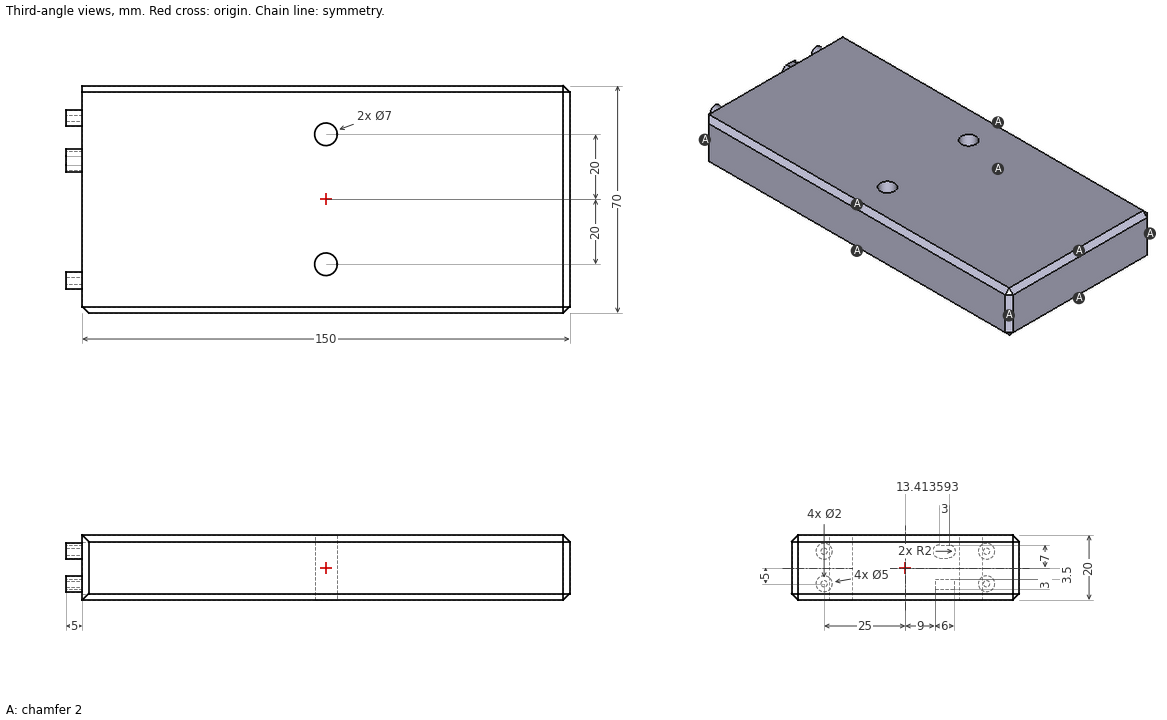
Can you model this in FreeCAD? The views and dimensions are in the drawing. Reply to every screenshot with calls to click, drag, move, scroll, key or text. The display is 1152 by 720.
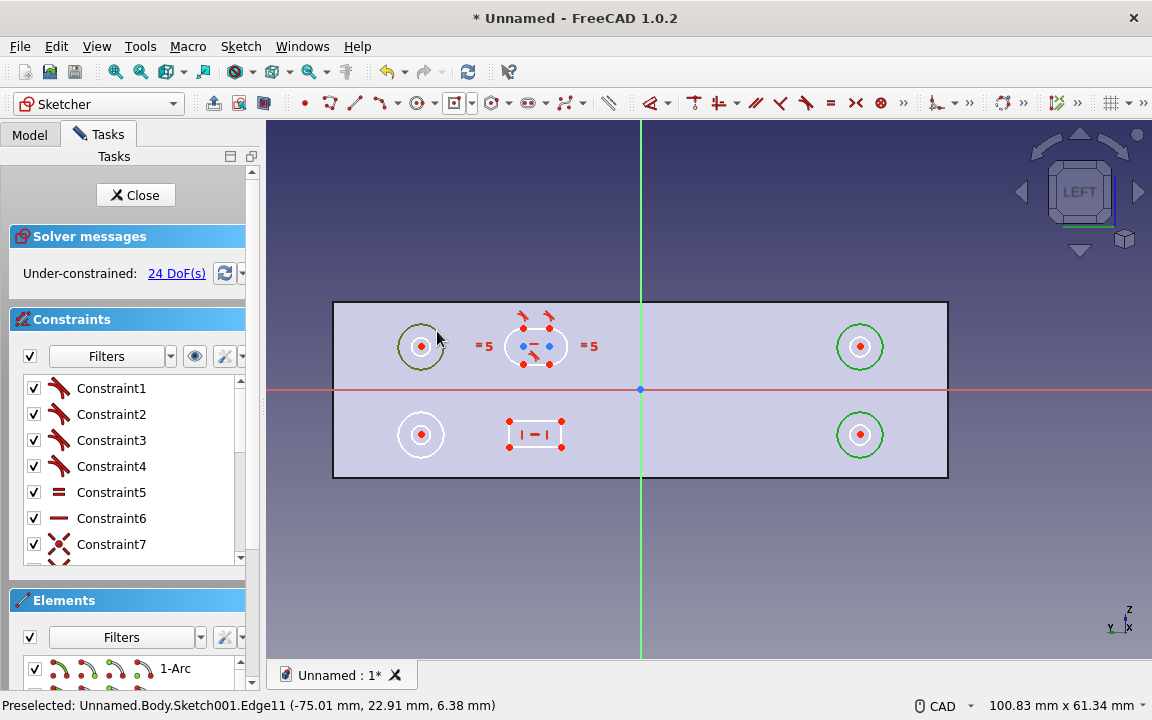
click(437, 419)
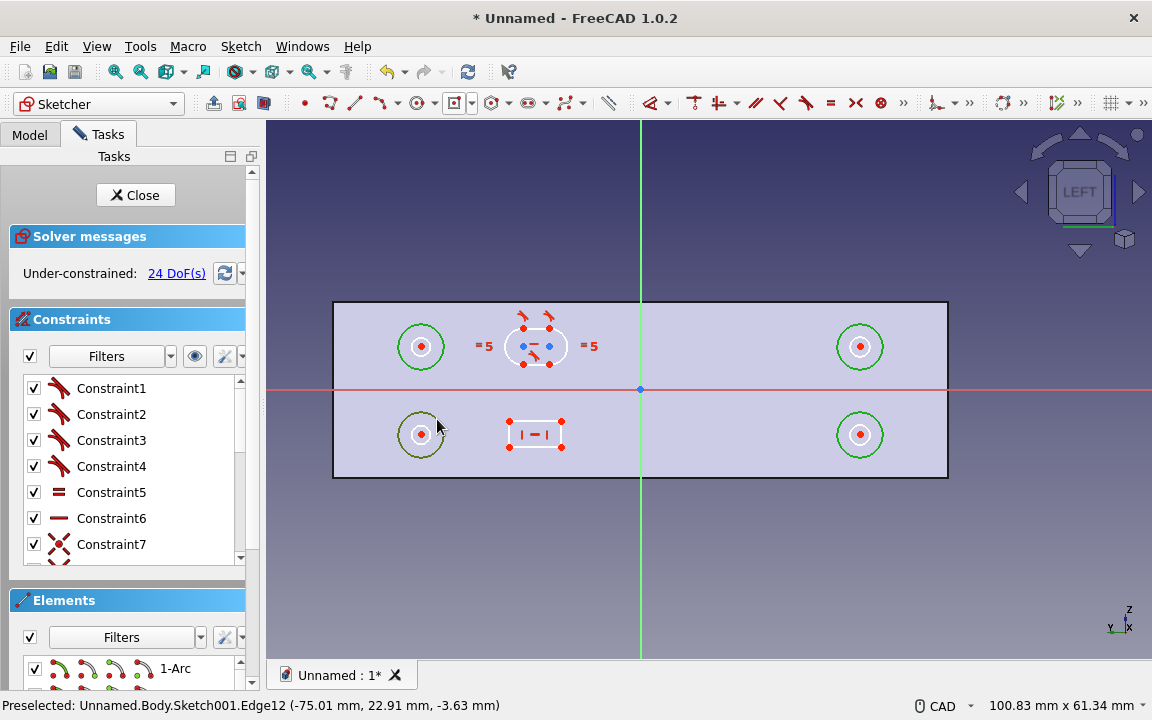
click(831, 104)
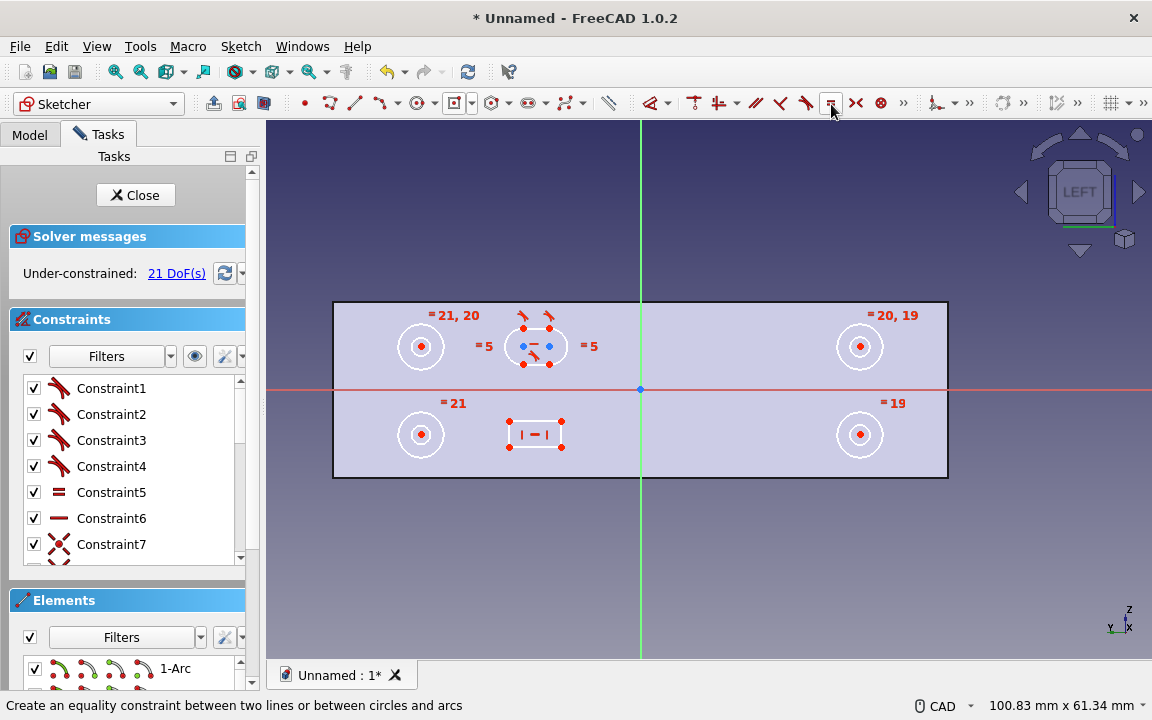
scroll(867, 428, up, 2)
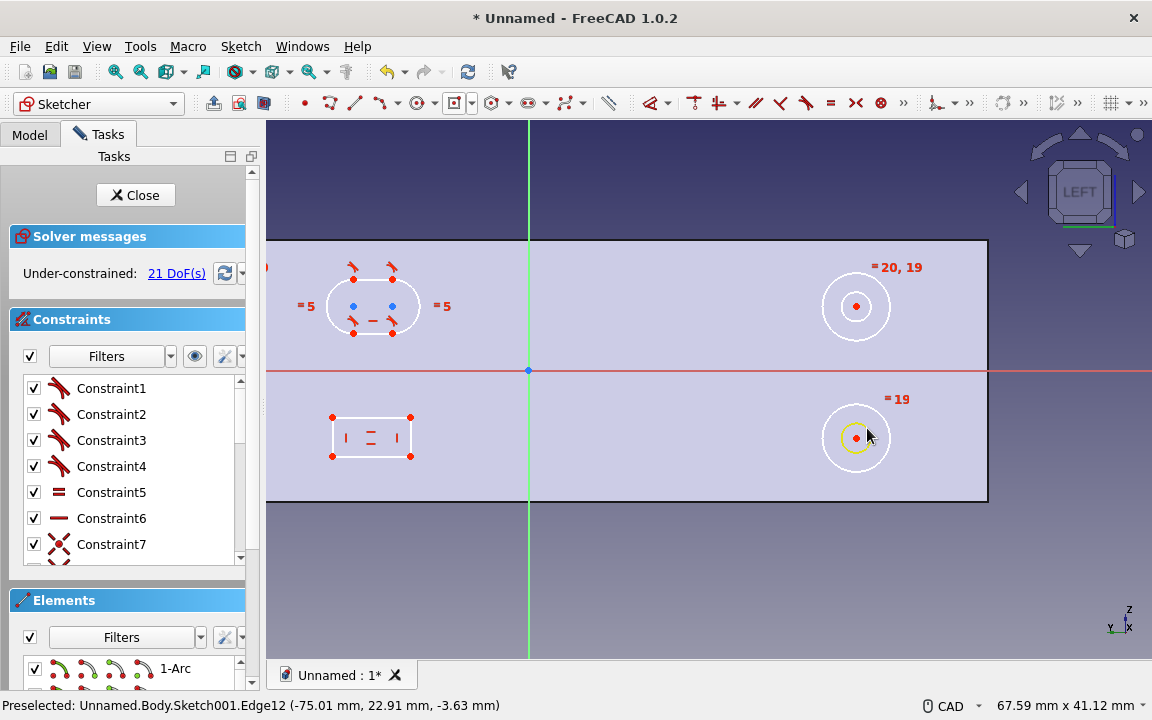
click(867, 428)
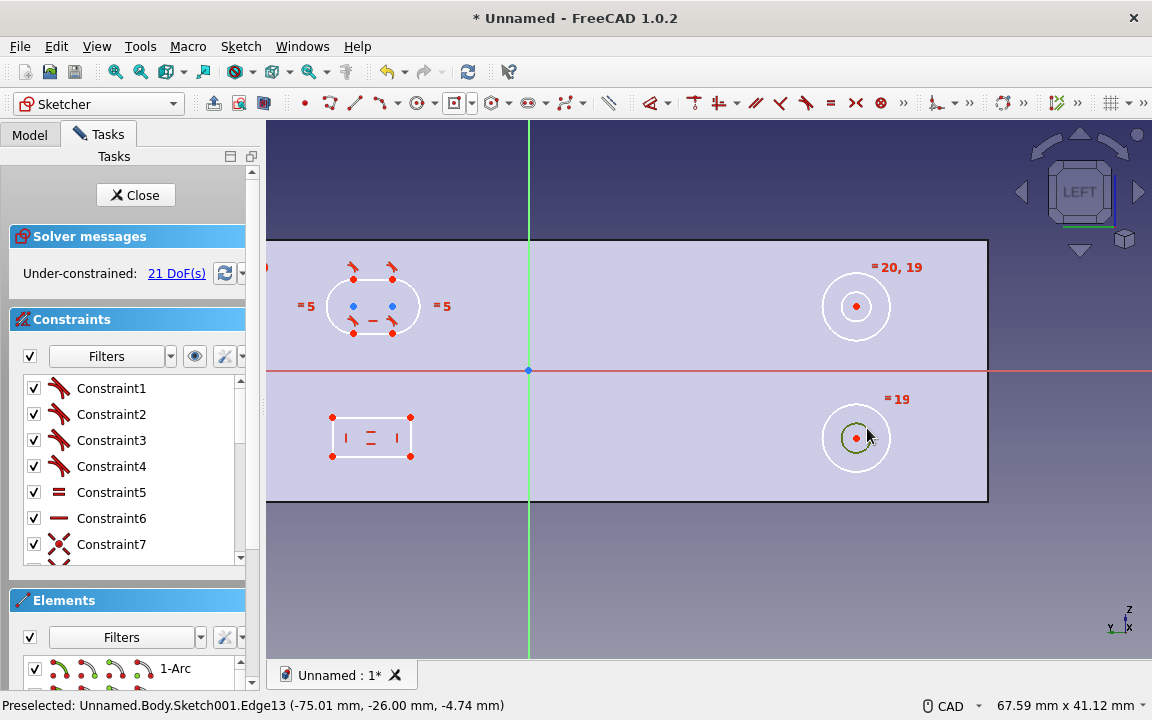
click(867, 297)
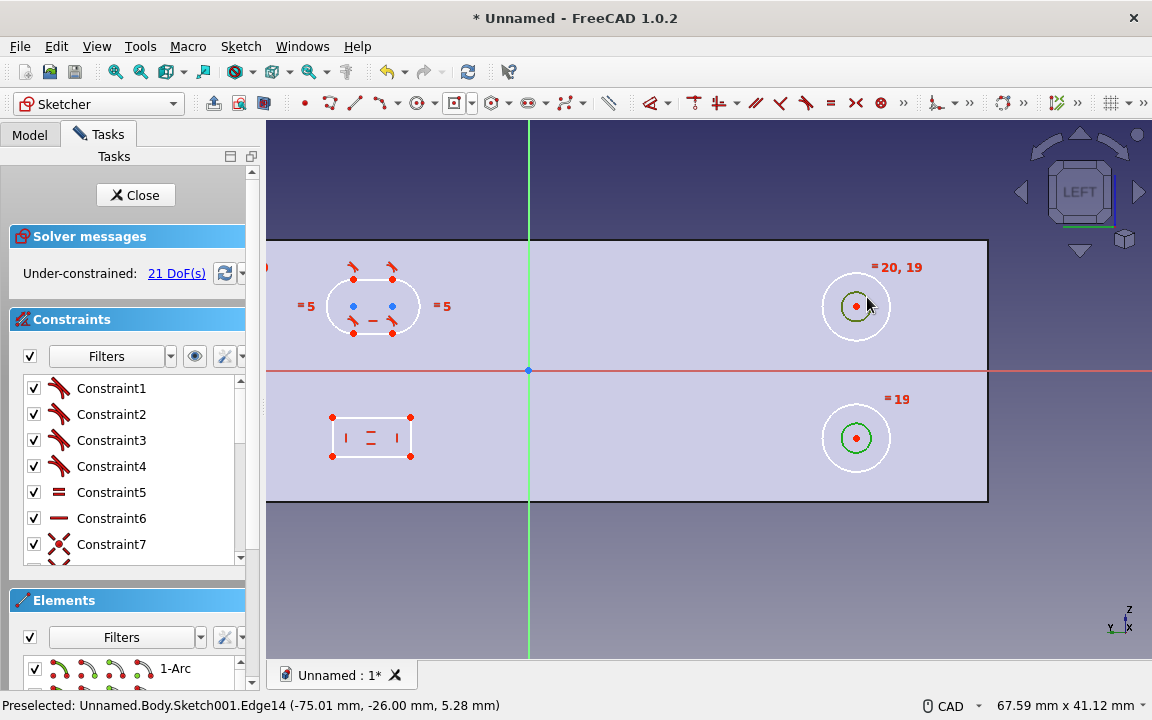
scroll(867, 428, down, 2)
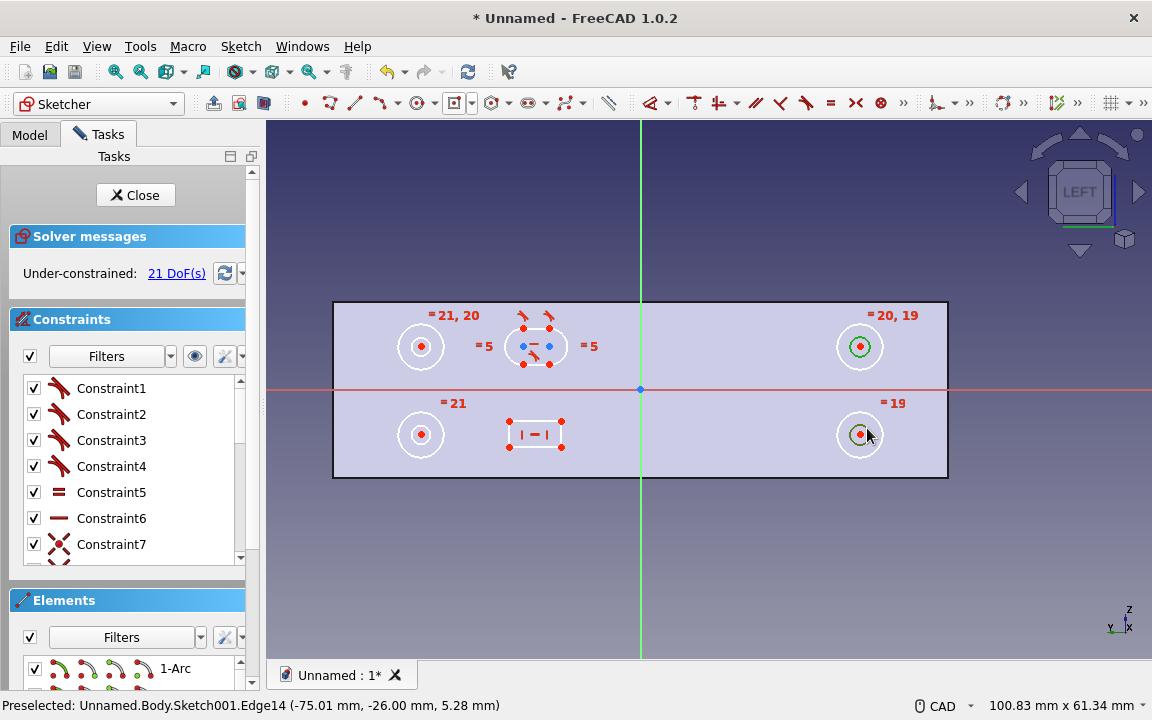
scroll(427, 340, up, 3)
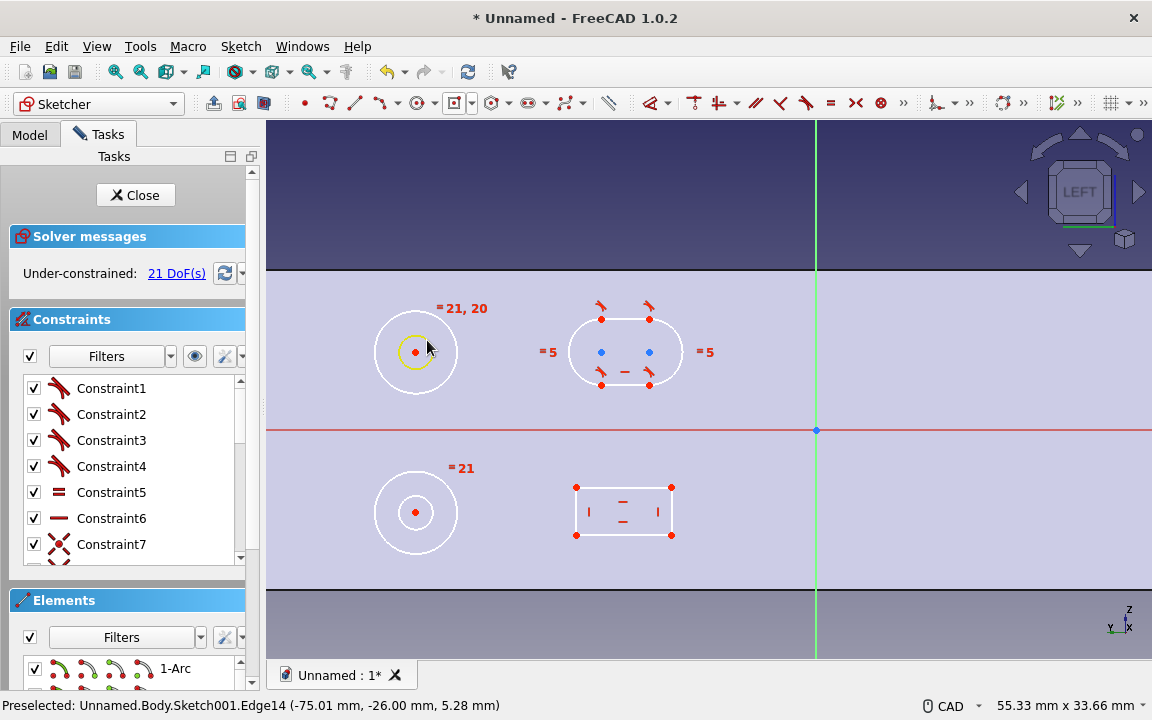
click(428, 341)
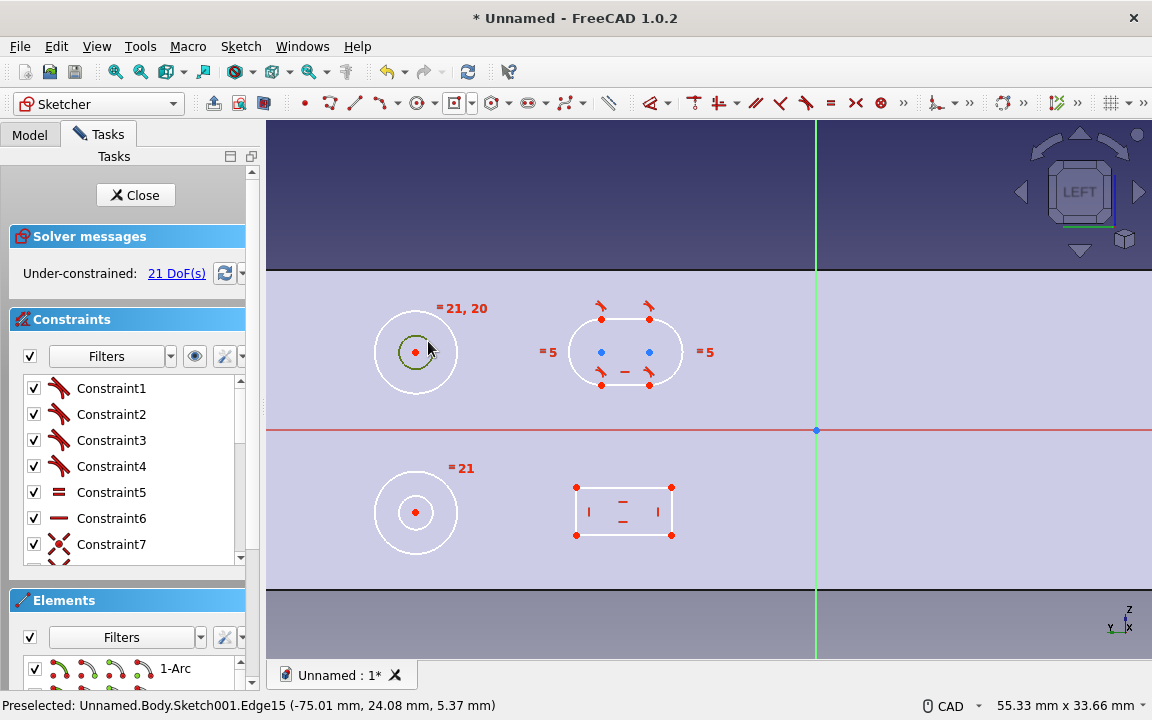
click(428, 501)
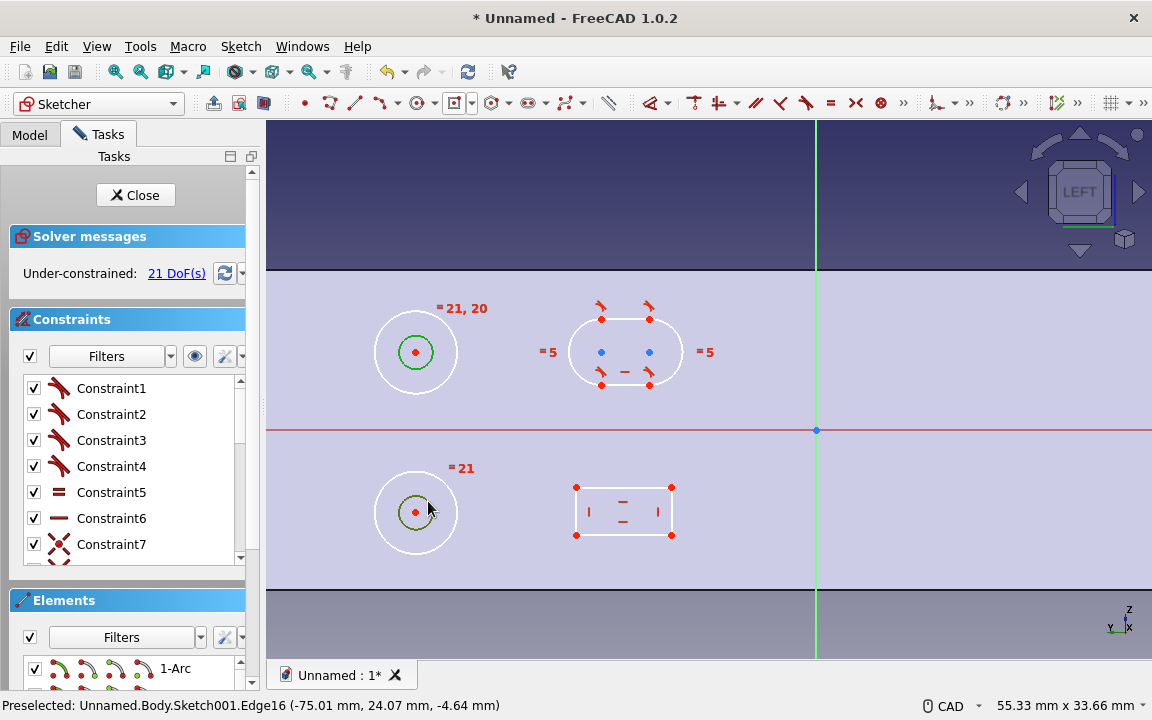
click(831, 104)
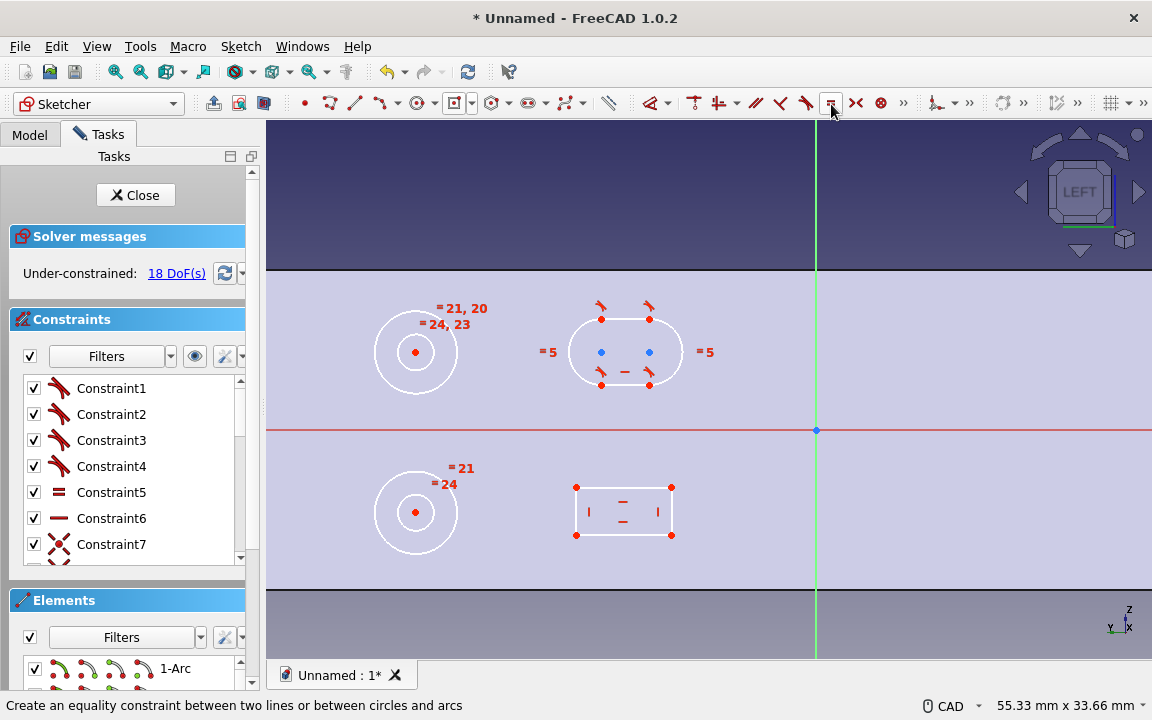
scroll(427, 340, down, 3)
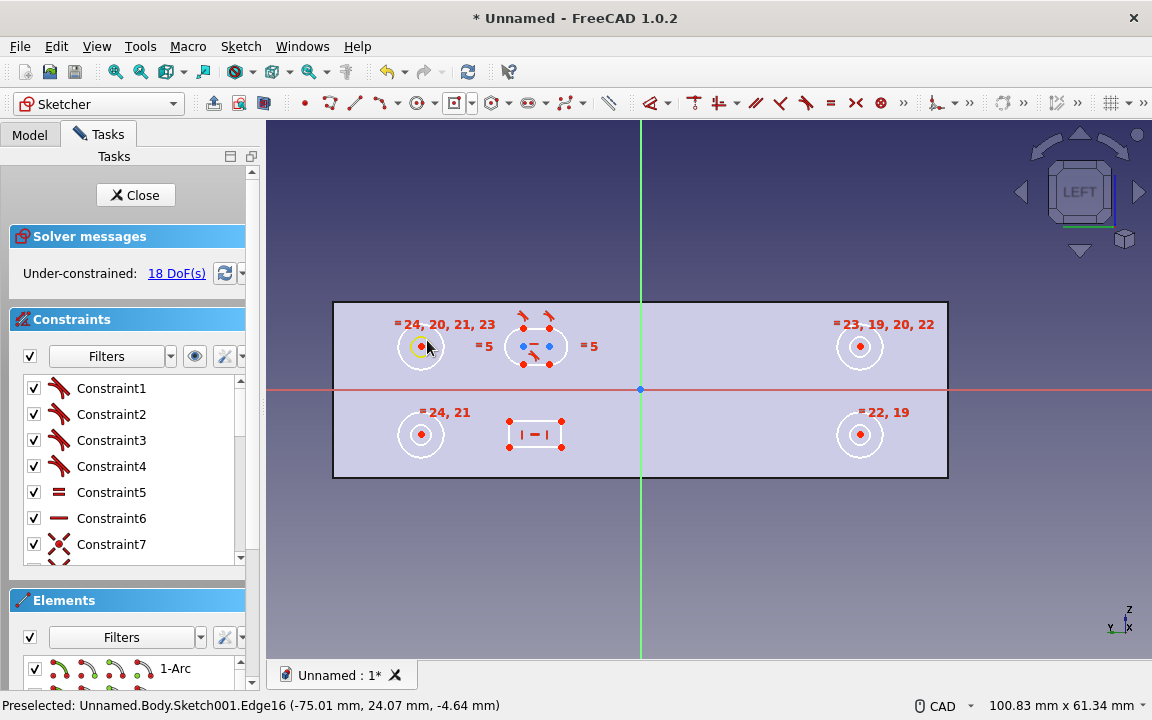
click(860, 435)